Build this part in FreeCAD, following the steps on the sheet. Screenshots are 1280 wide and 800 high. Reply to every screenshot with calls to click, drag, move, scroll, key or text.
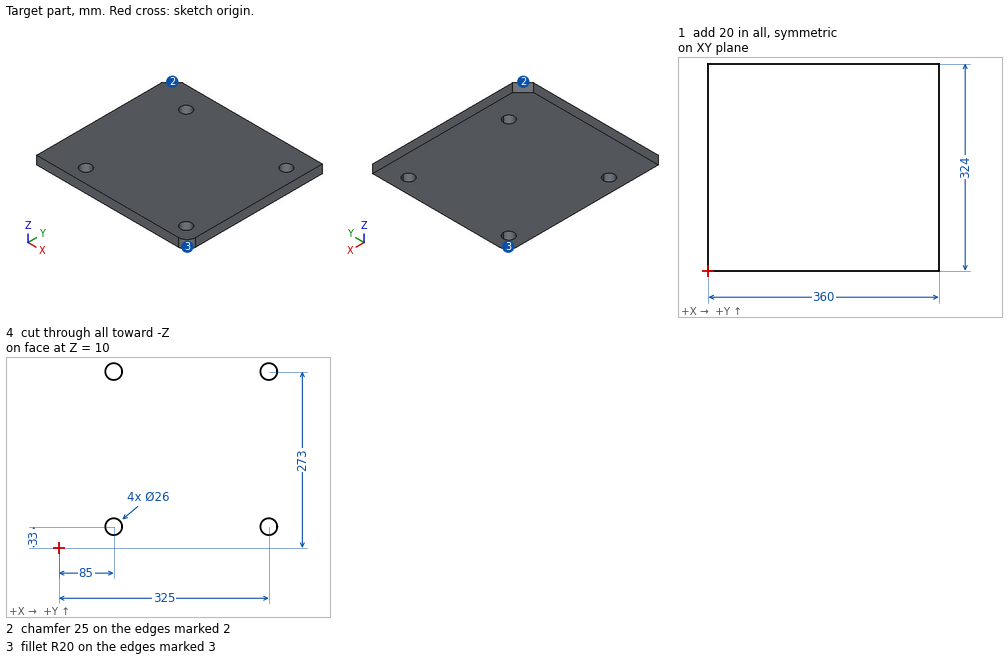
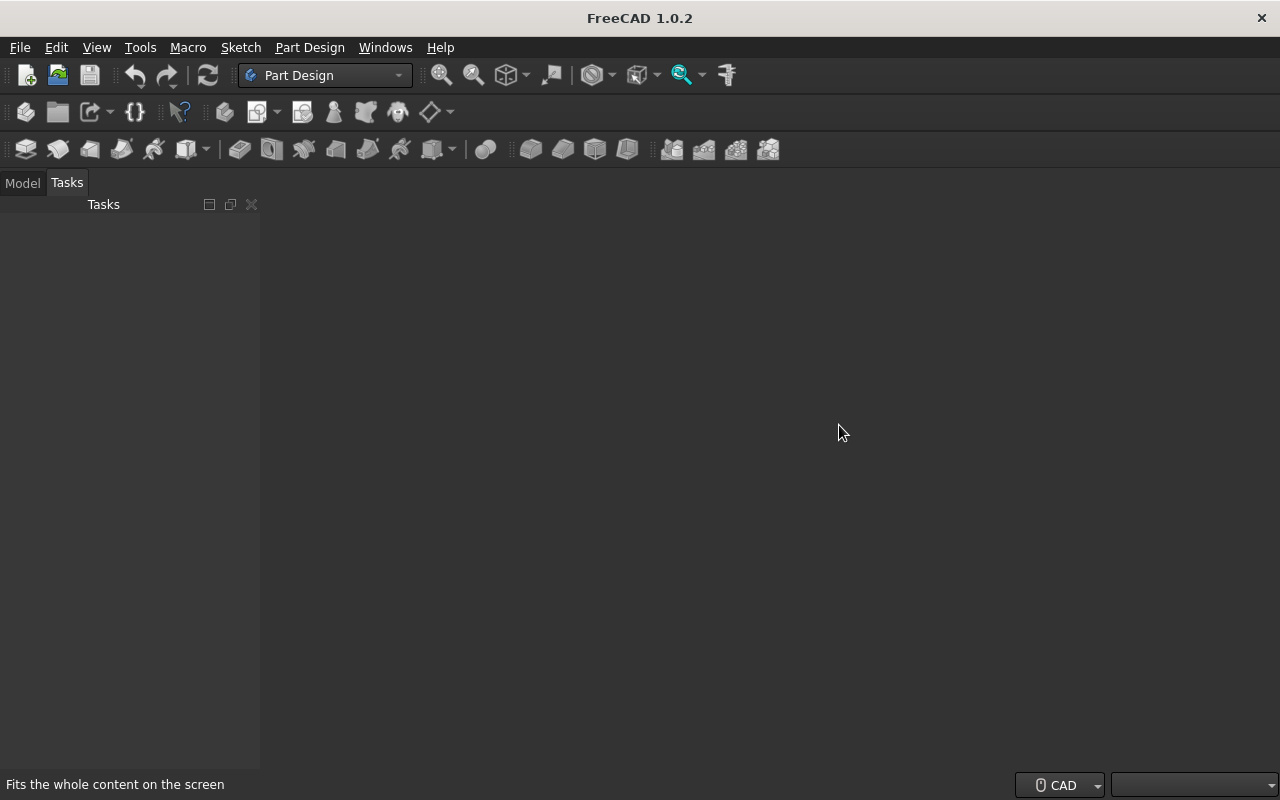
click(26, 76)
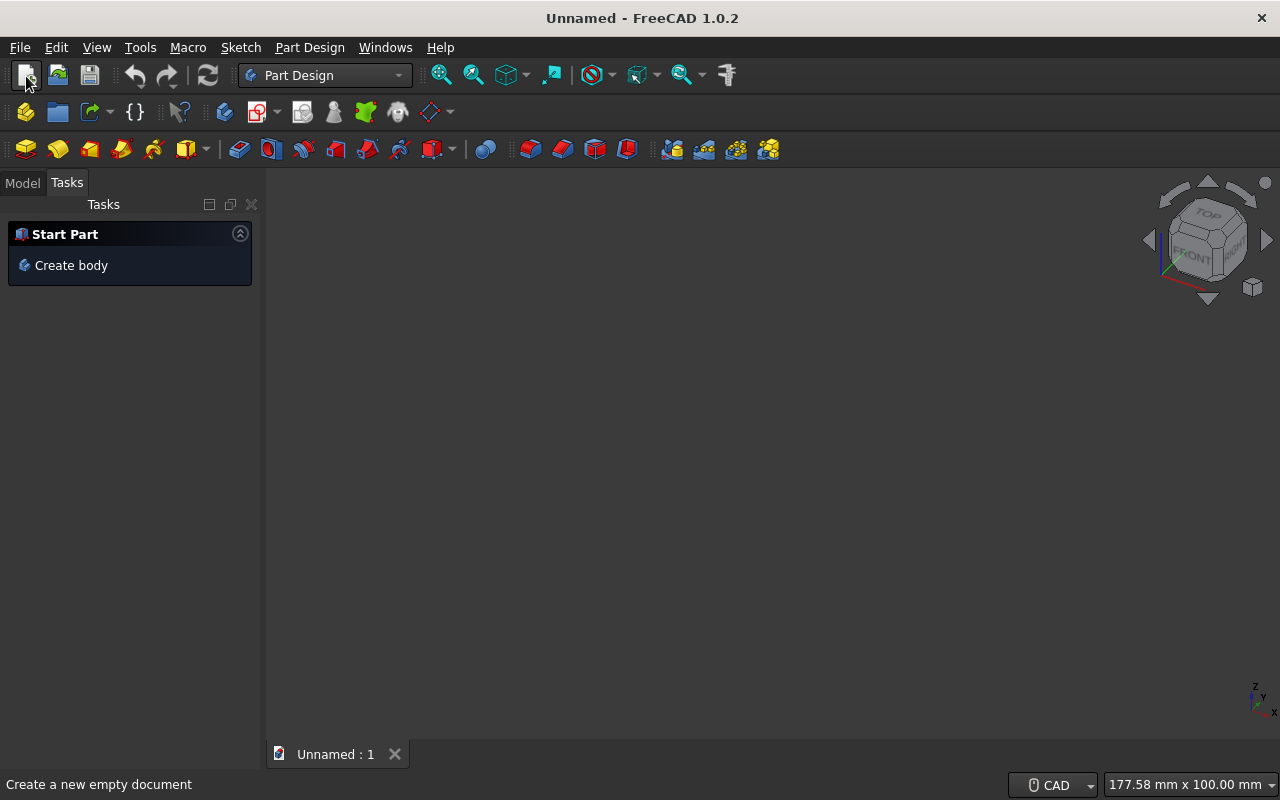
click(258, 112)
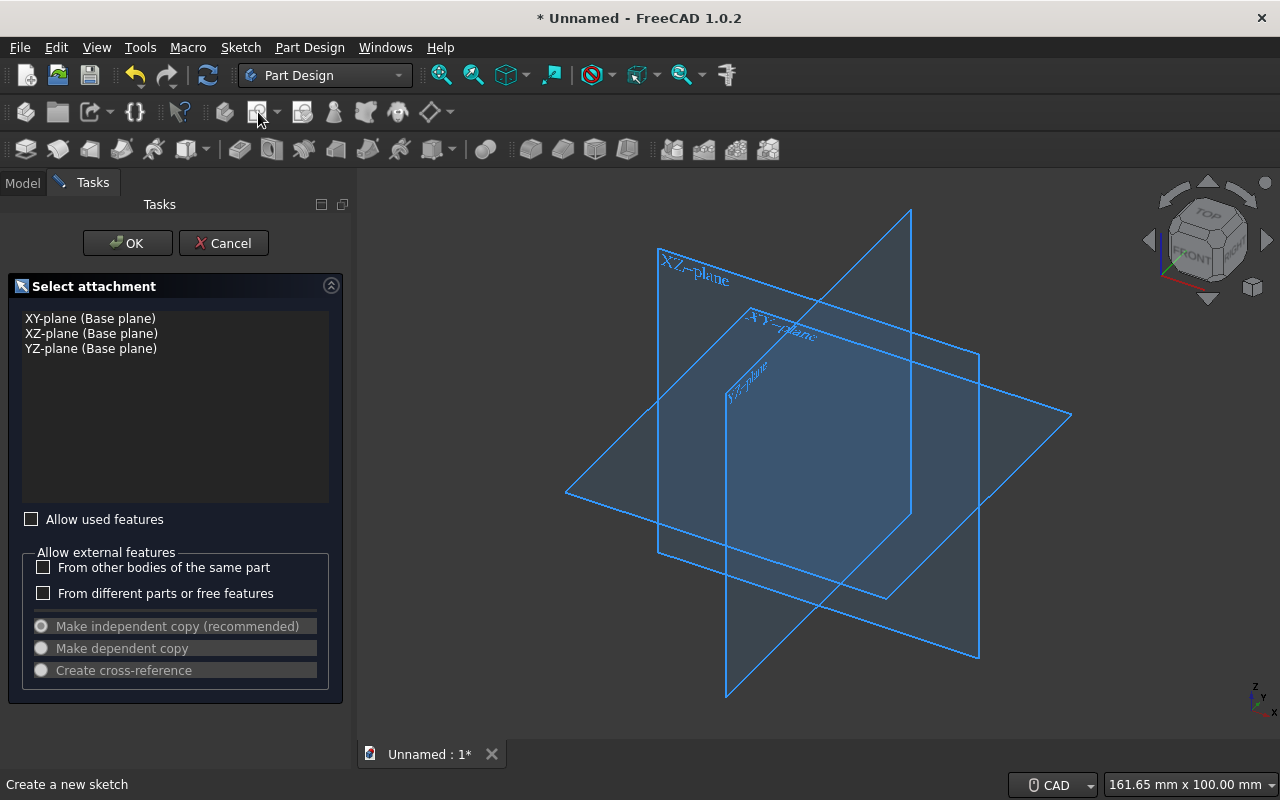
click(82, 318)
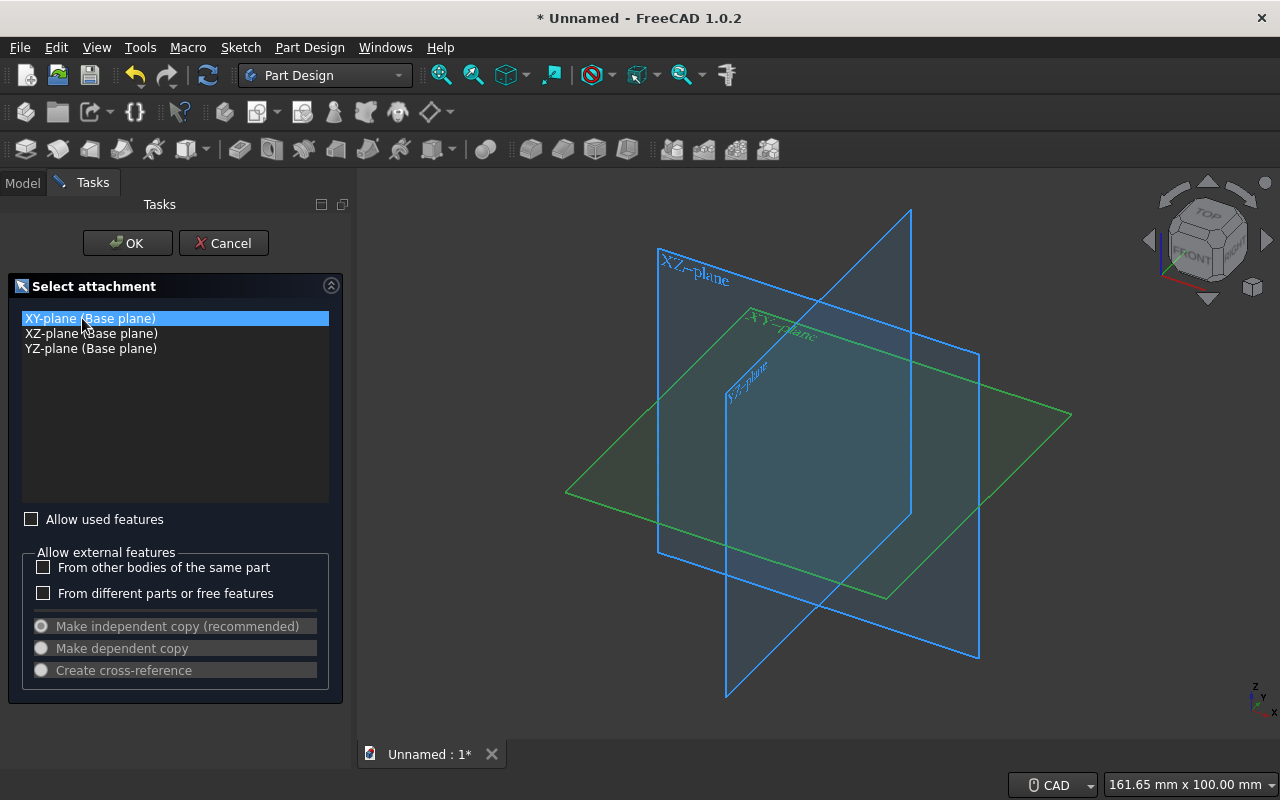
click(128, 243)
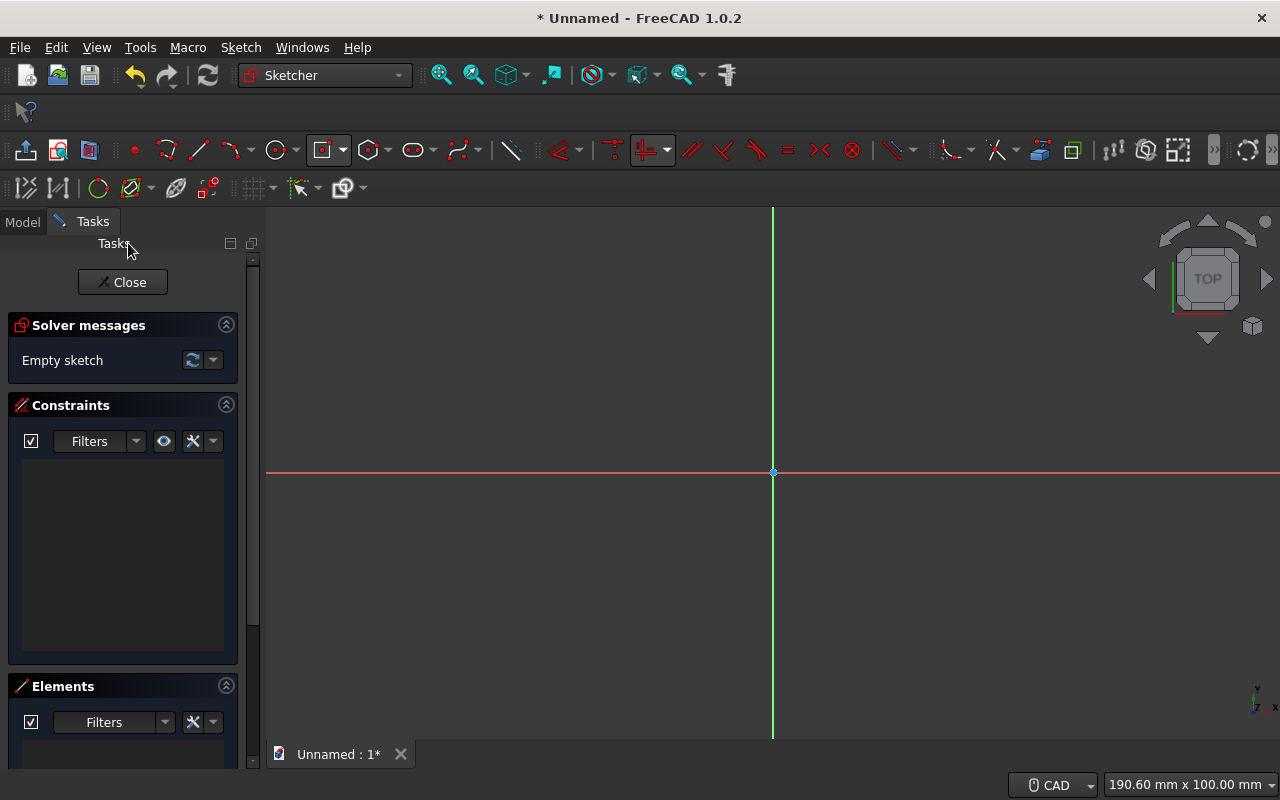
scroll(445, 691, down, 8)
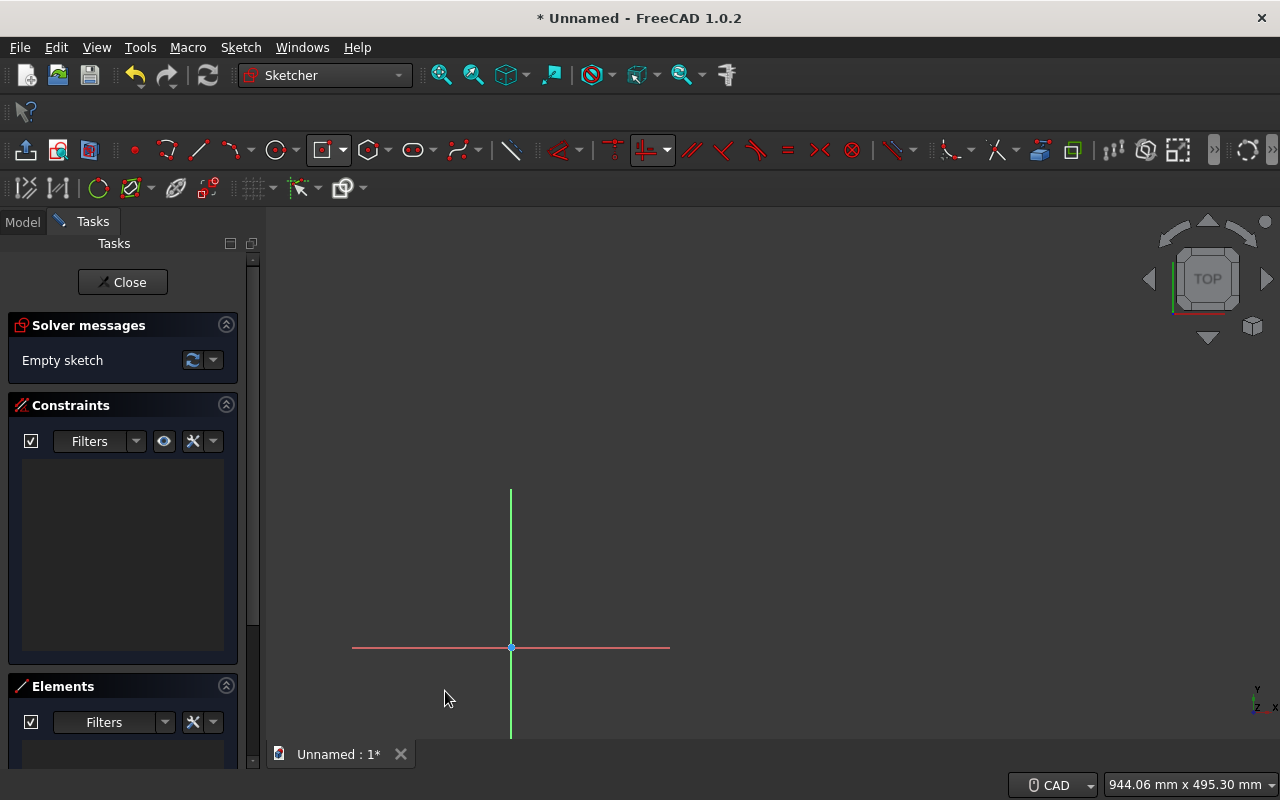
key(g)
key(r)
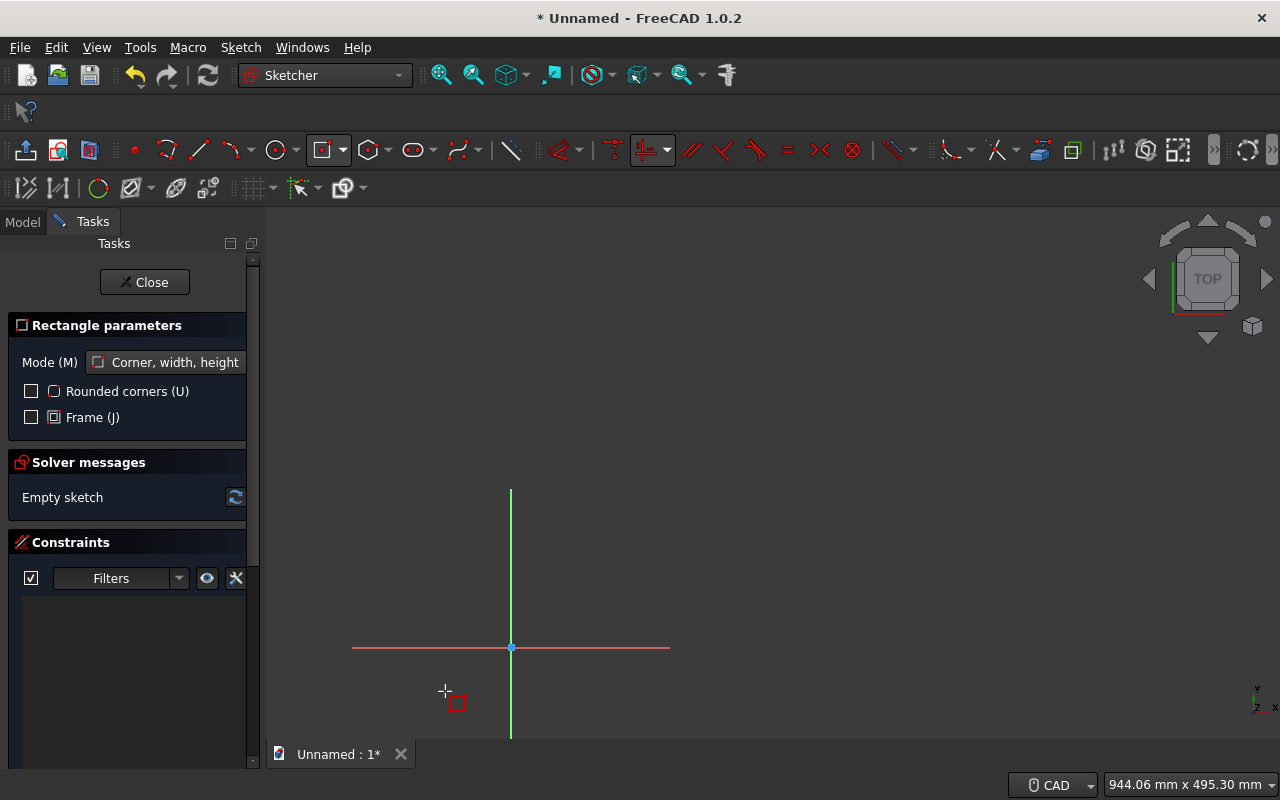
click(511, 648)
click(898, 300)
key(Escape)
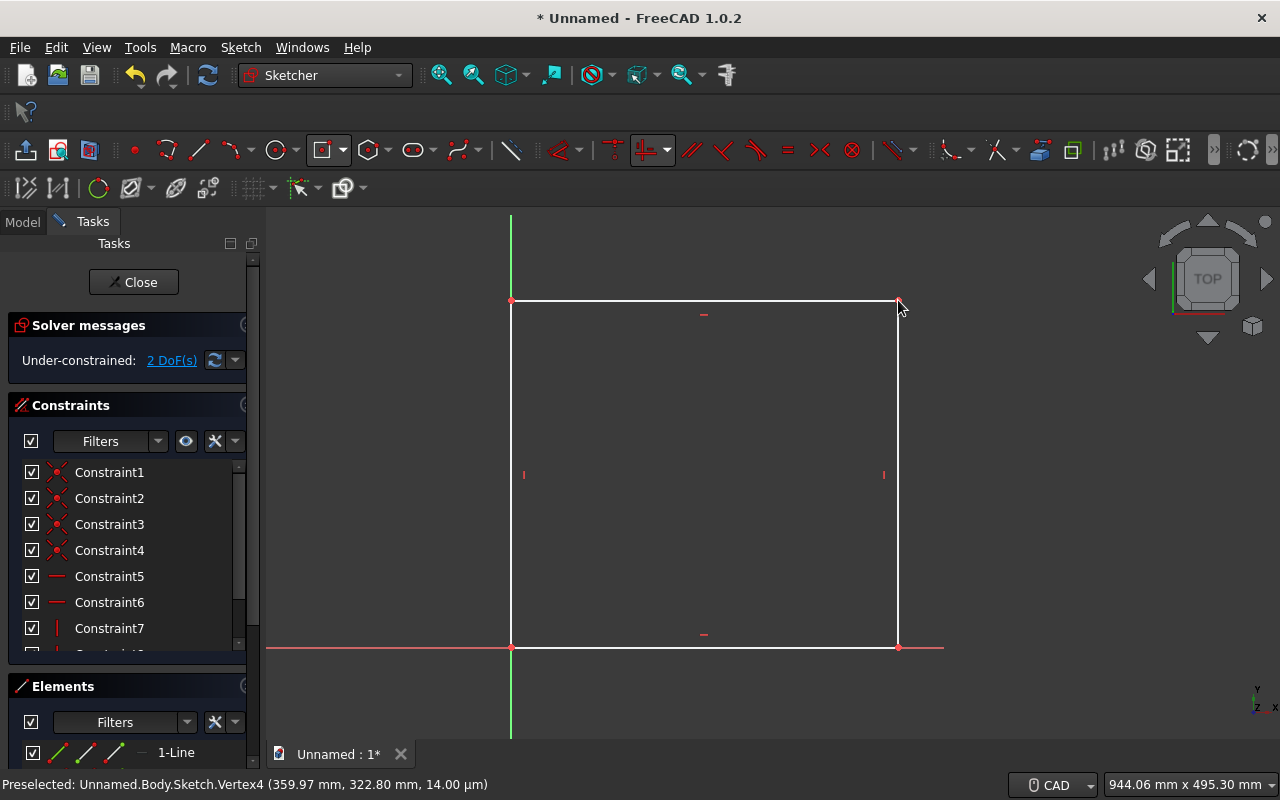
click(558, 150)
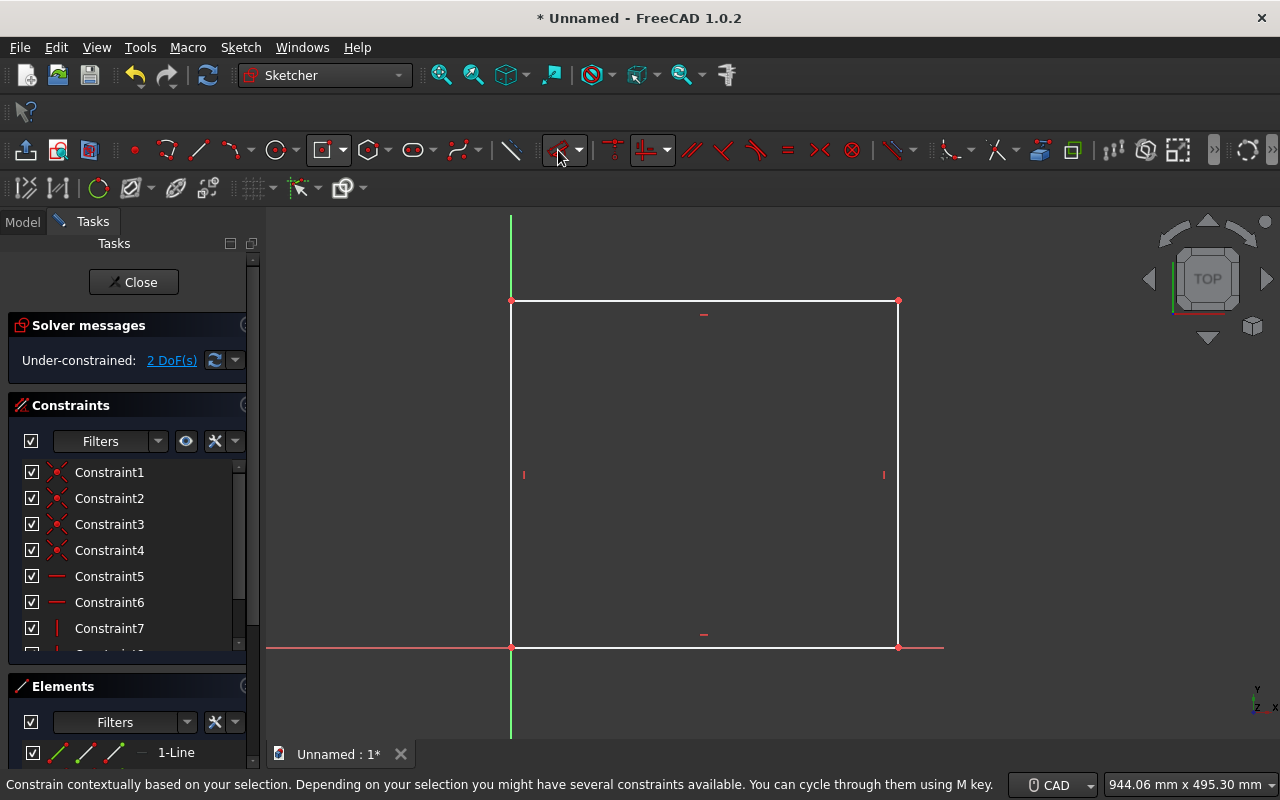
click(627, 648)
click(705, 682)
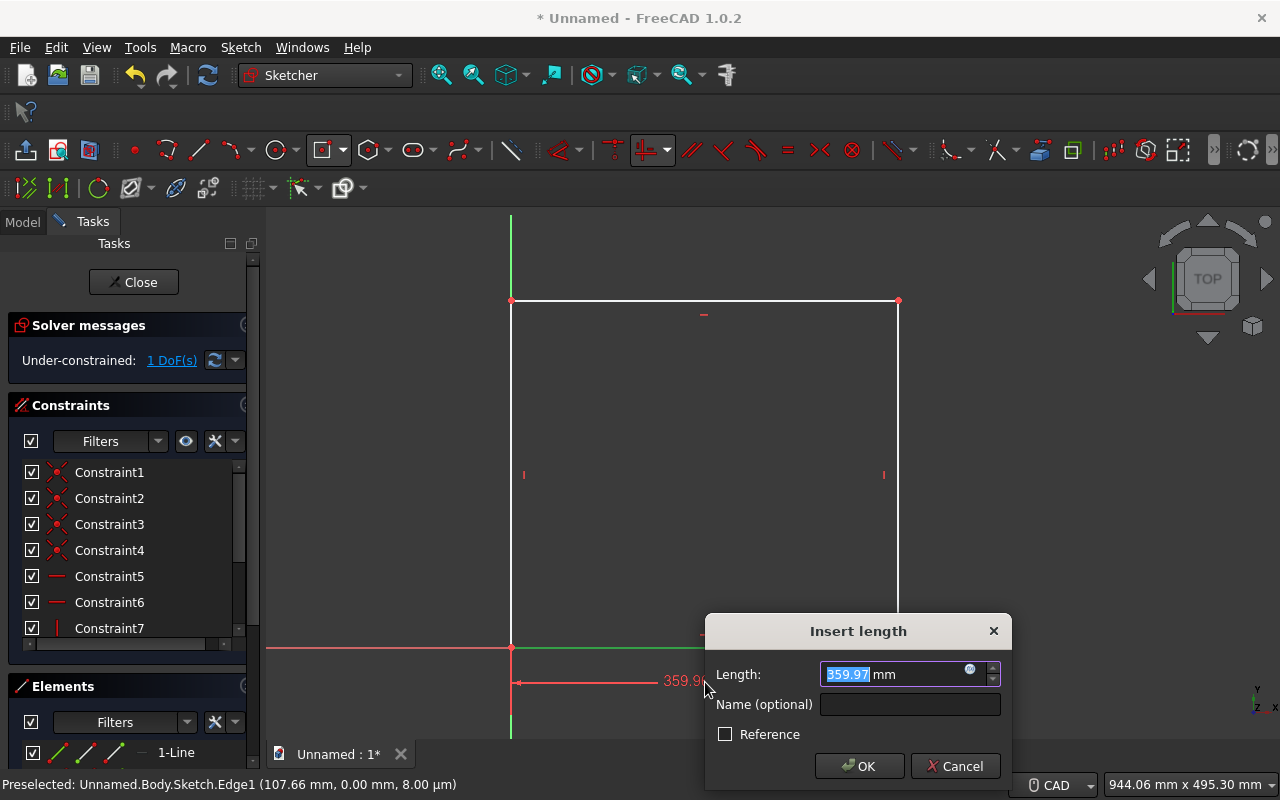
text(360)
key(Return)